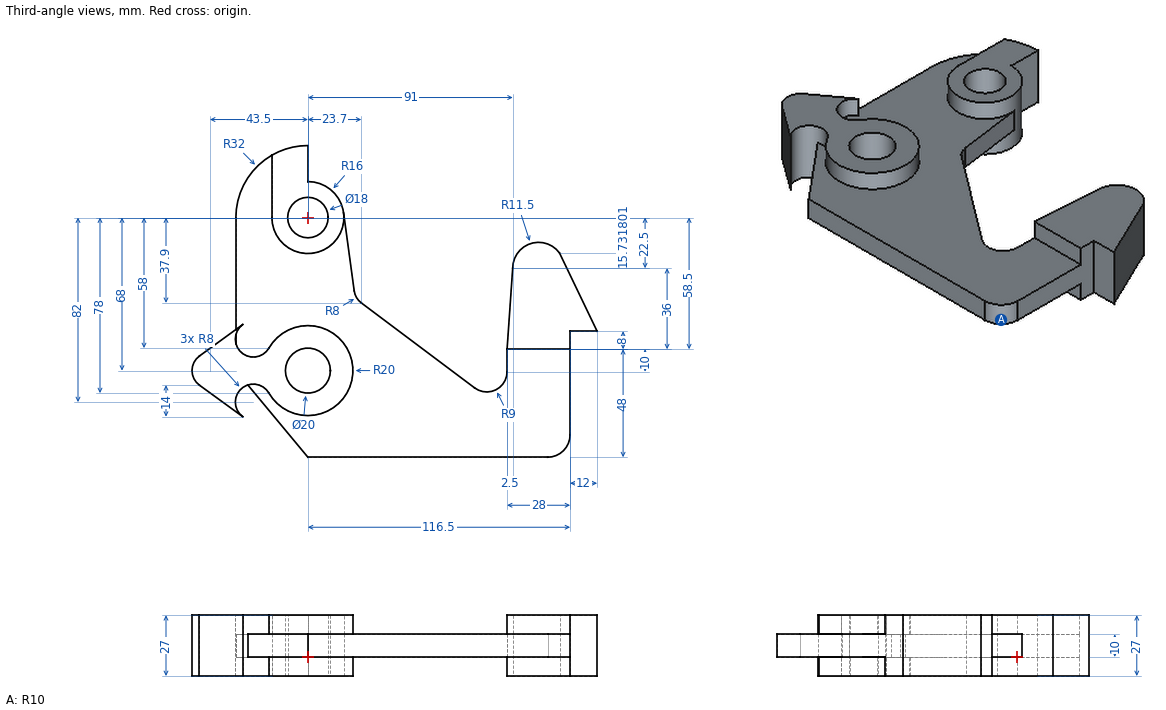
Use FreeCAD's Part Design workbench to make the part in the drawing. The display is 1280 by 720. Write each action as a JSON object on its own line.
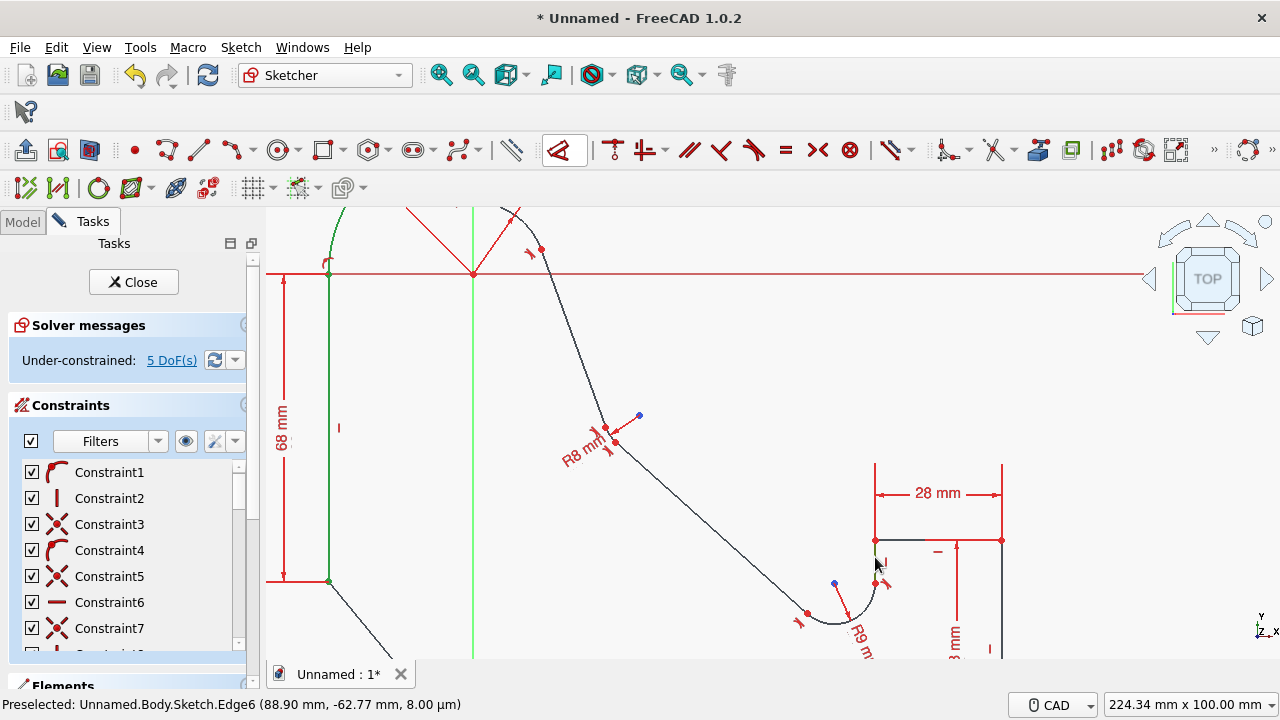
{"action": "key", "text": "i"}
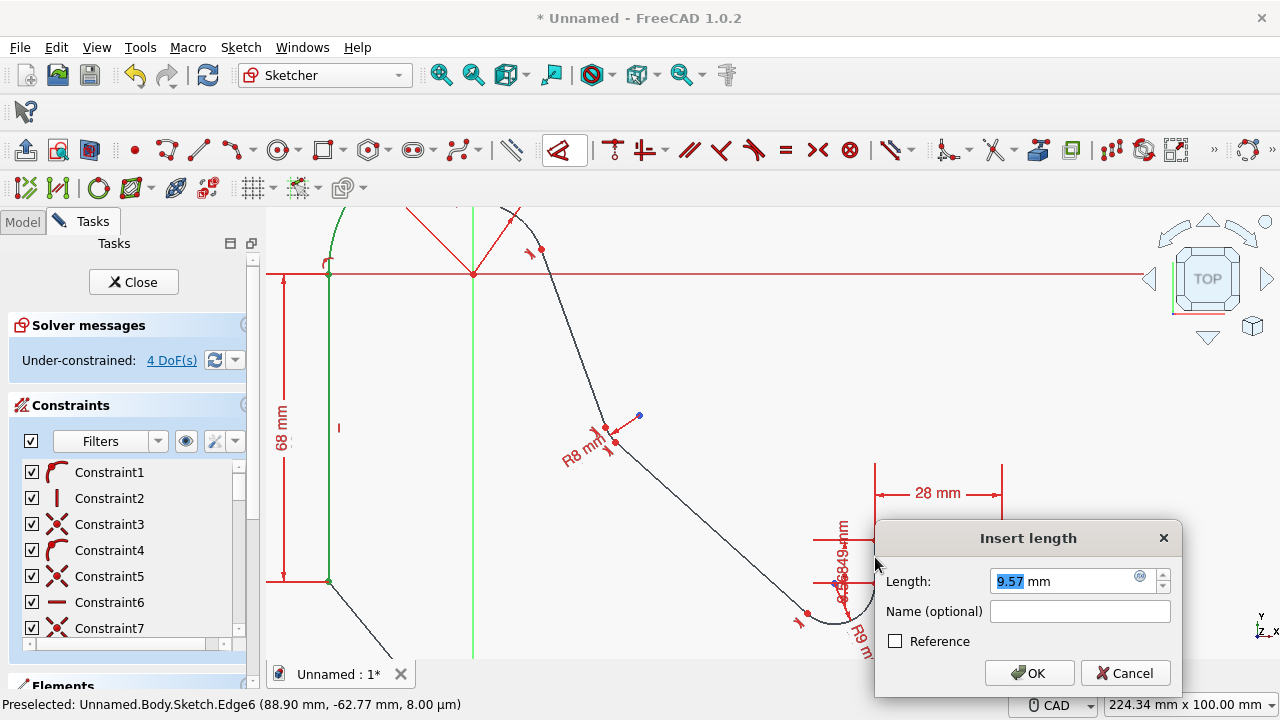
{"action": "type", "text": "10"}
{"action": "key", "text": "Return"}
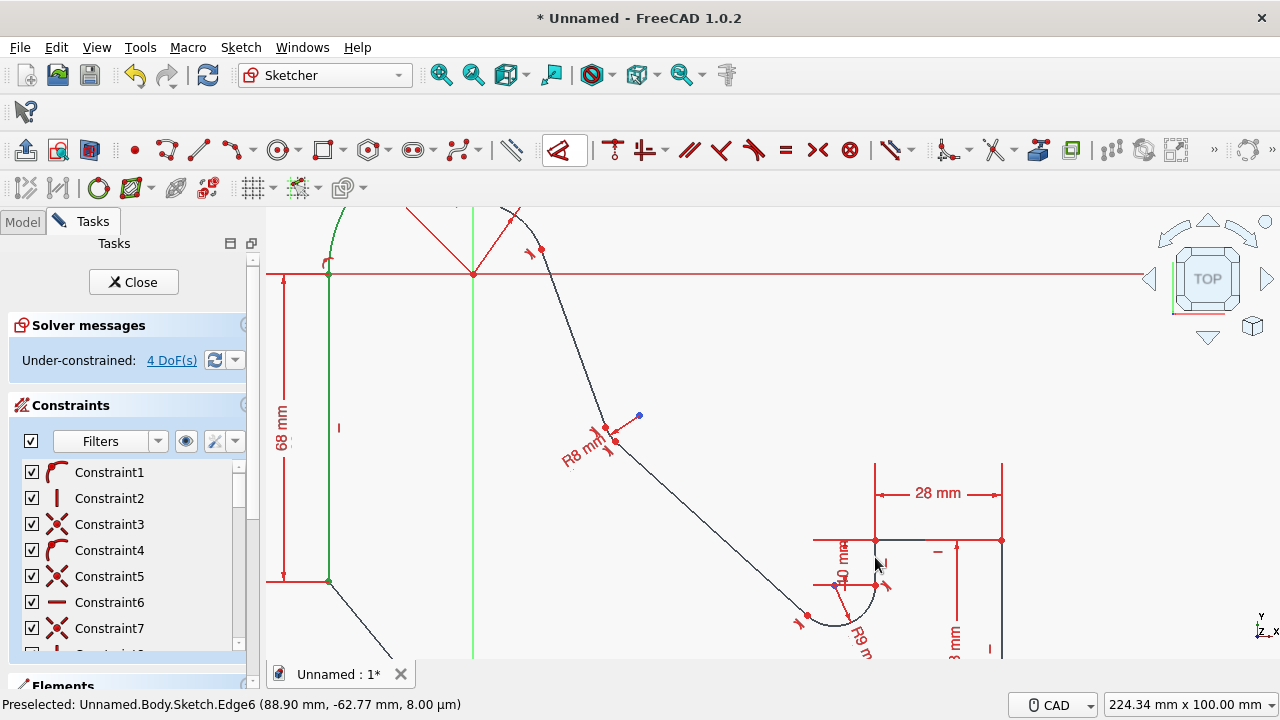
{"action": "scroll", "coordinate": [737, 425], "scroll_direction": "down", "scroll_amount": 4}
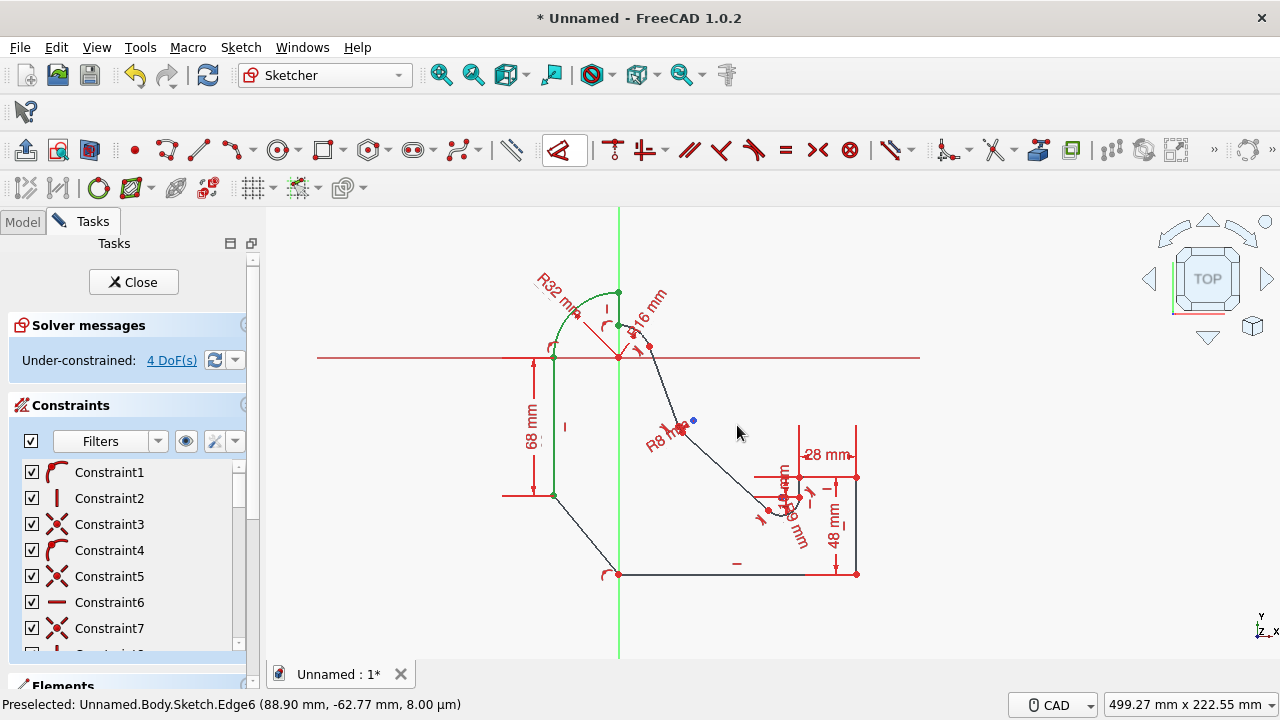
{"action": "left_click", "coordinate": [690, 575]}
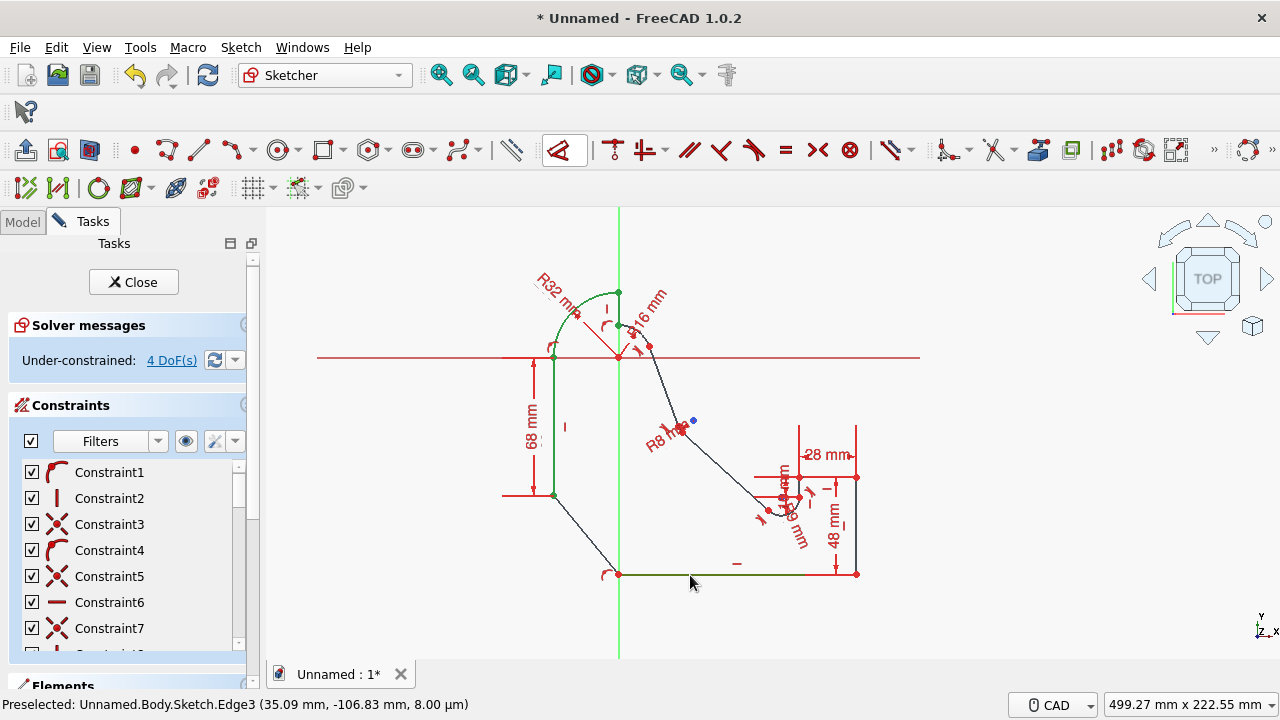
{"action": "left_click", "coordinate": [582, 150]}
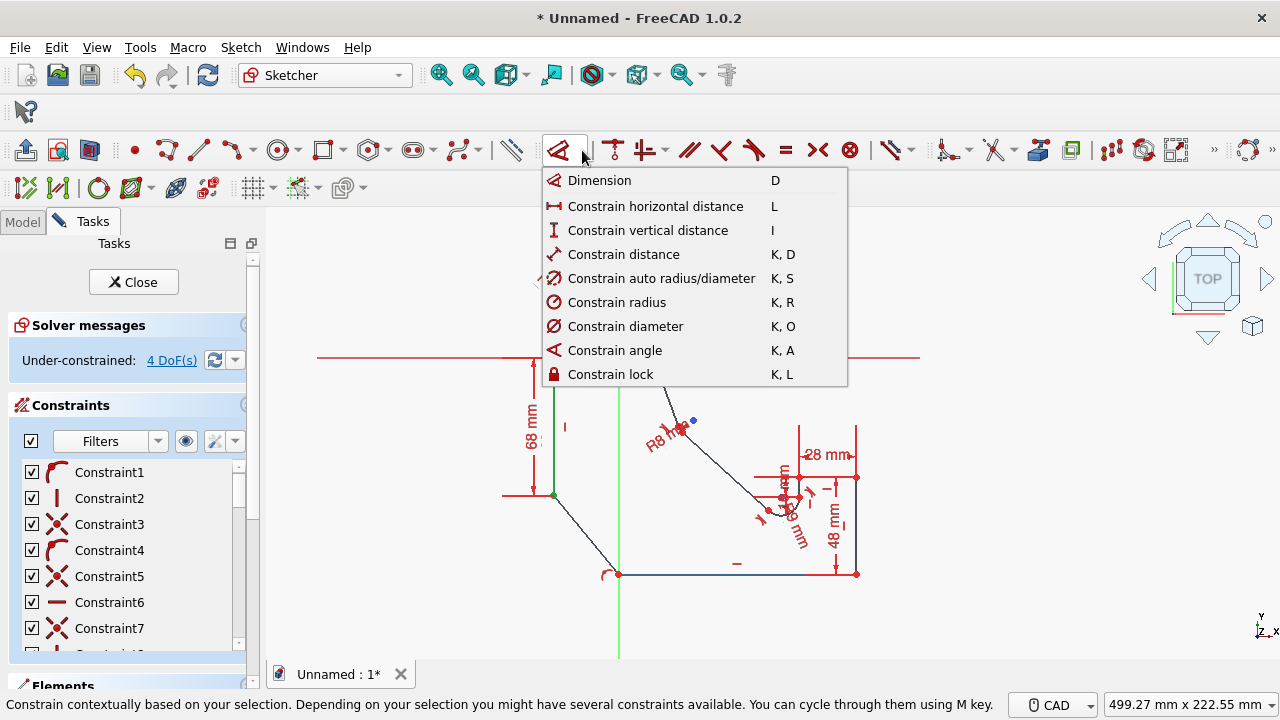
{"action": "left_click", "coordinate": [695, 206]}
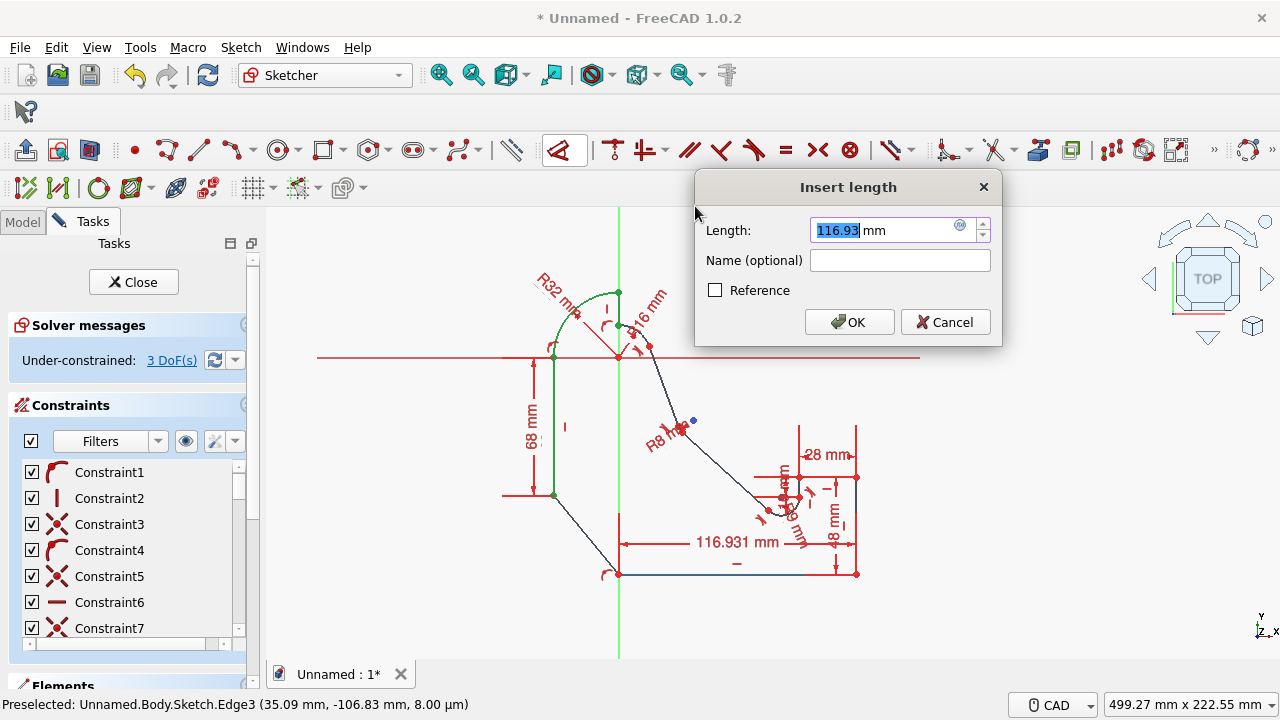
{"action": "type", "text": "116.5"}
{"action": "key", "text": "Return"}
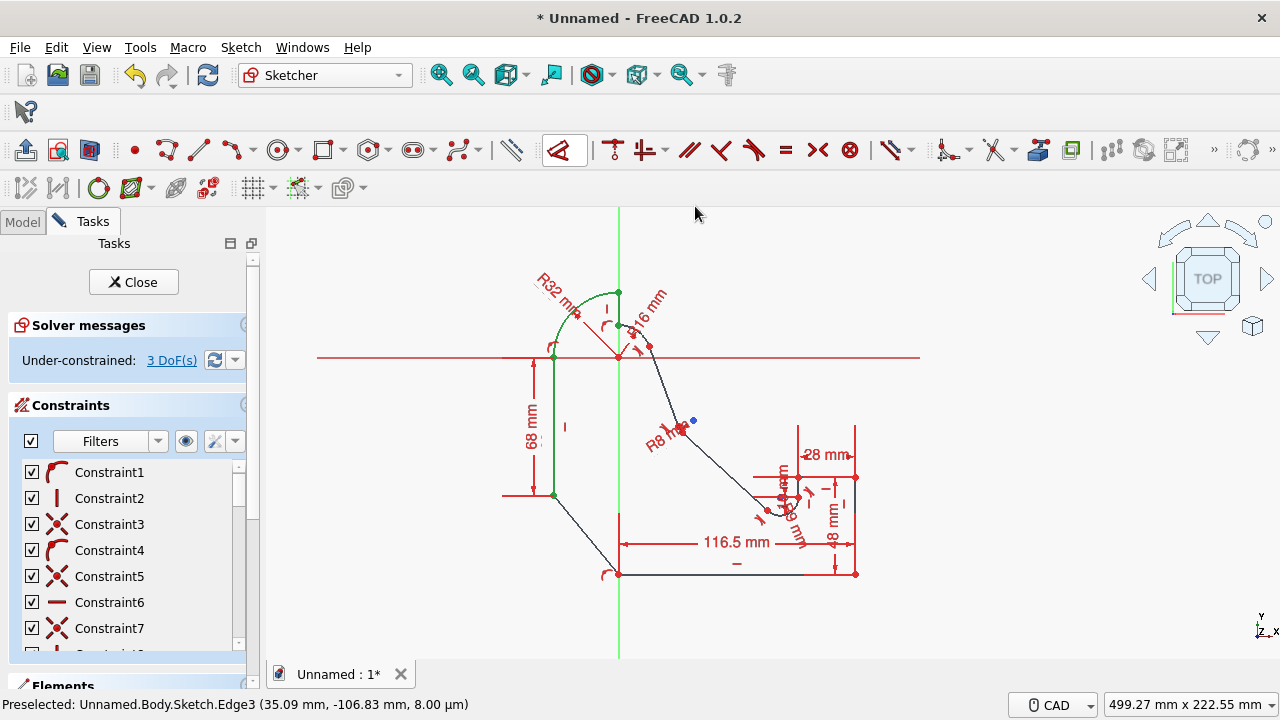
{"action": "left_click", "coordinate": [855, 477]}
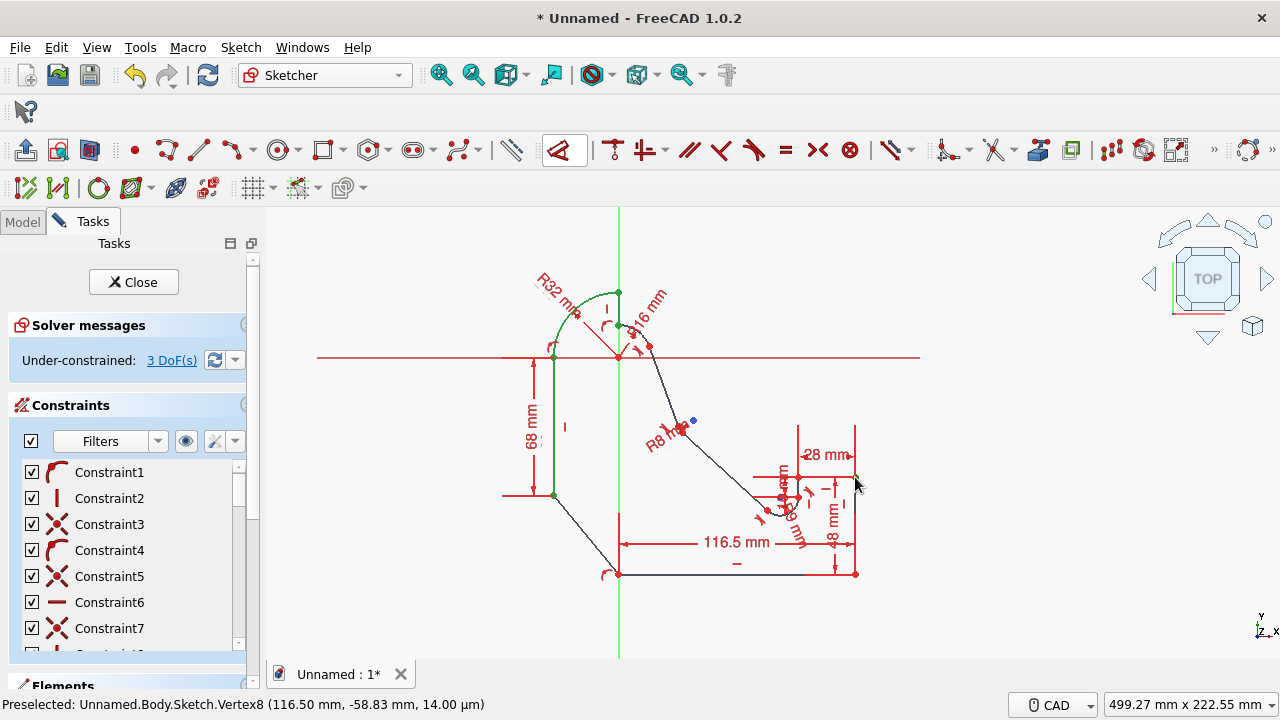
{"action": "key", "text": "i"}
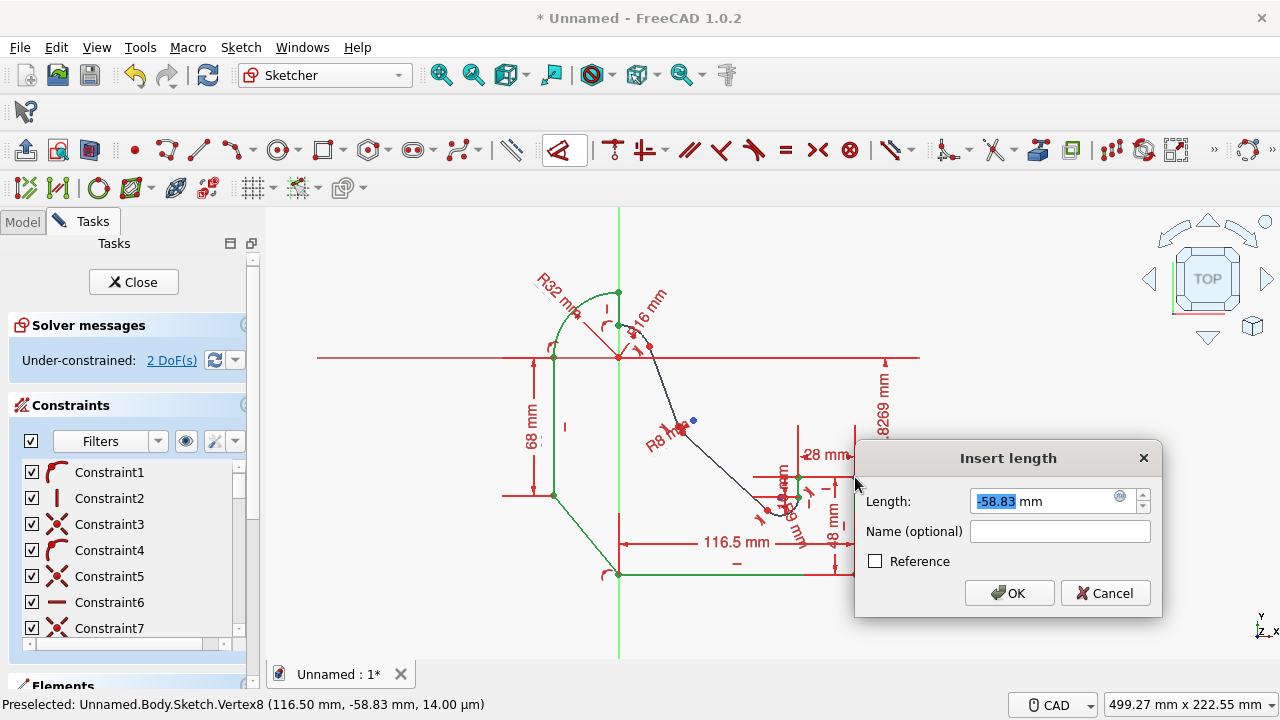
{"action": "type", "text": "-58.5"}
{"action": "key", "text": "Return"}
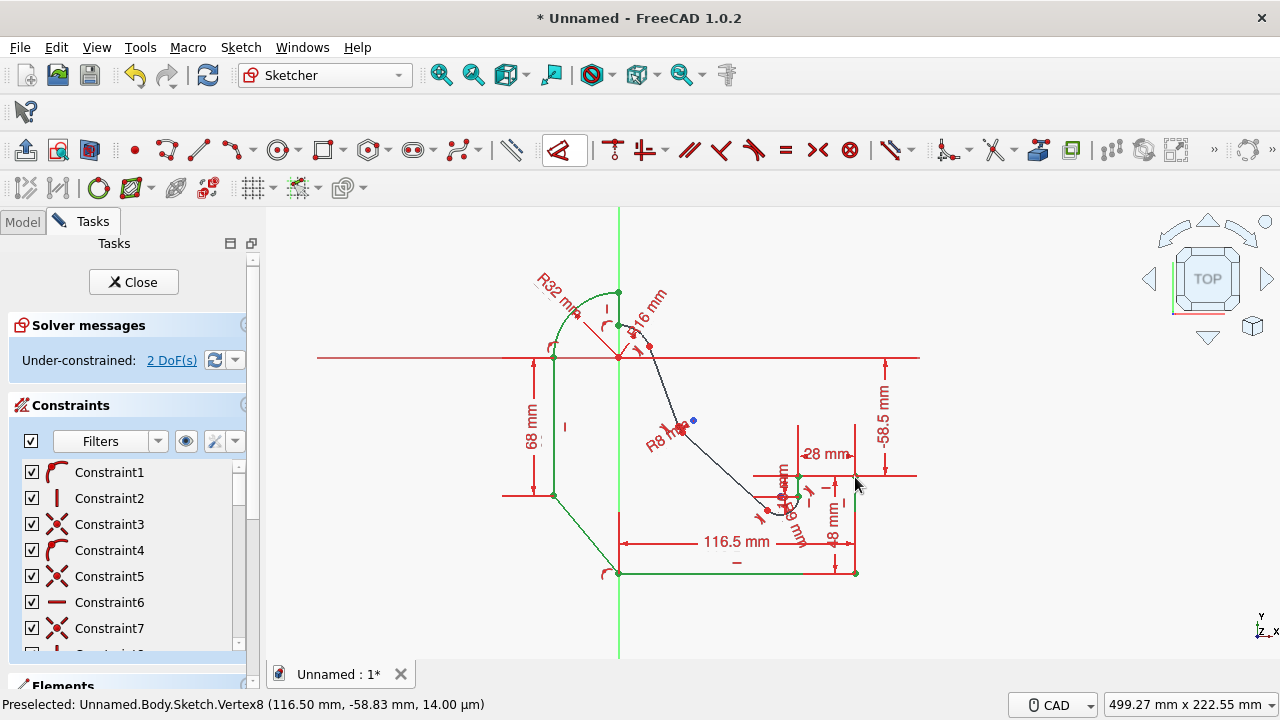
{"action": "scroll", "coordinate": [683, 433], "scroll_direction": "up", "scroll_amount": 3}